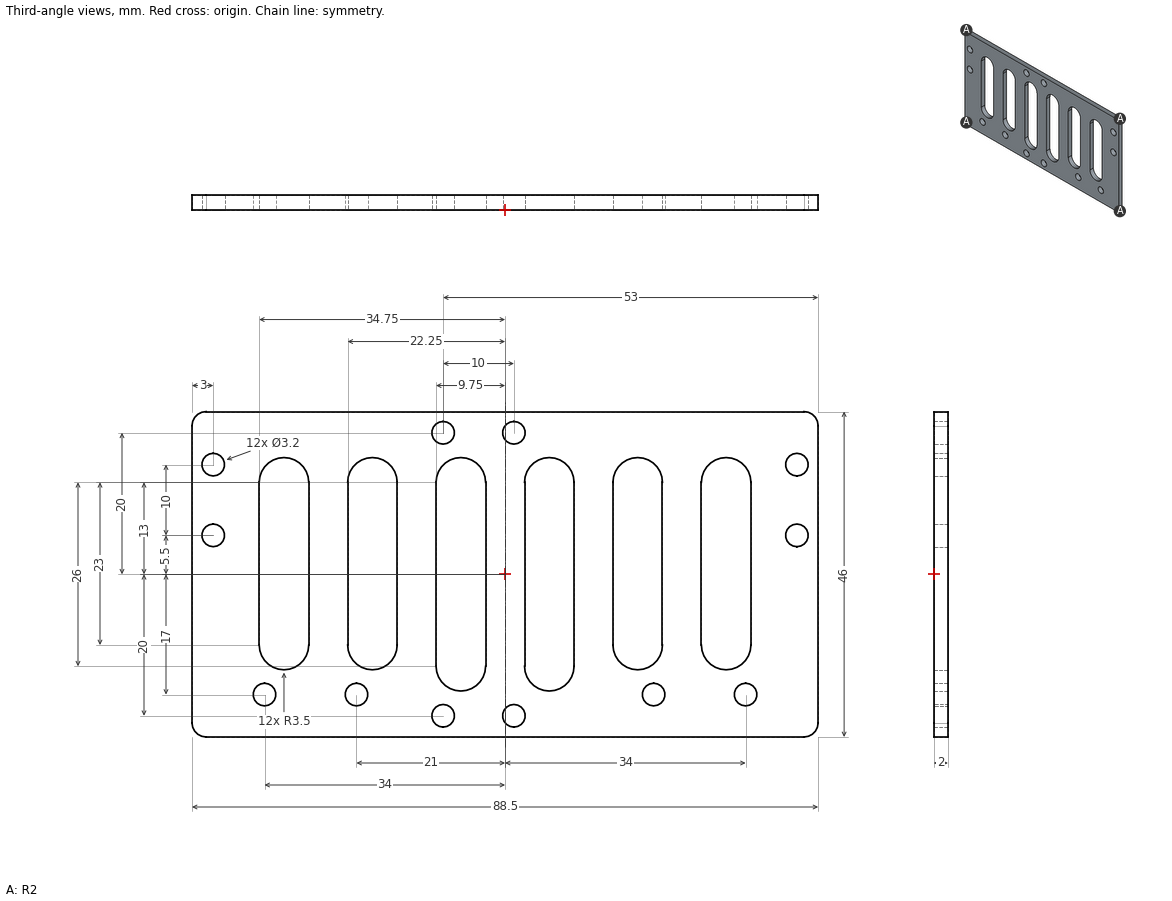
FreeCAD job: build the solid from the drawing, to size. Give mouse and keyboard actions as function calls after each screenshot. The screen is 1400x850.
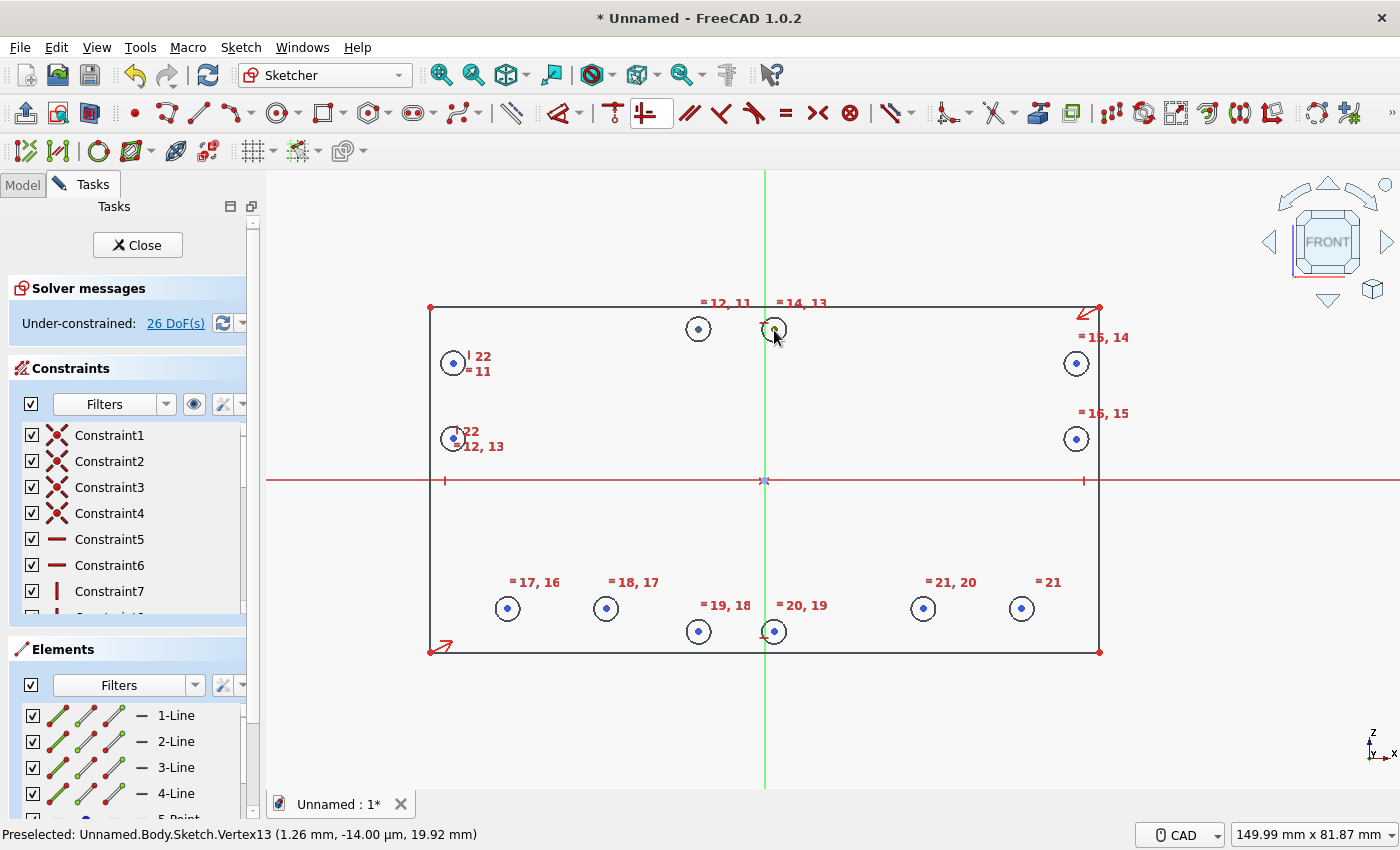
key(h)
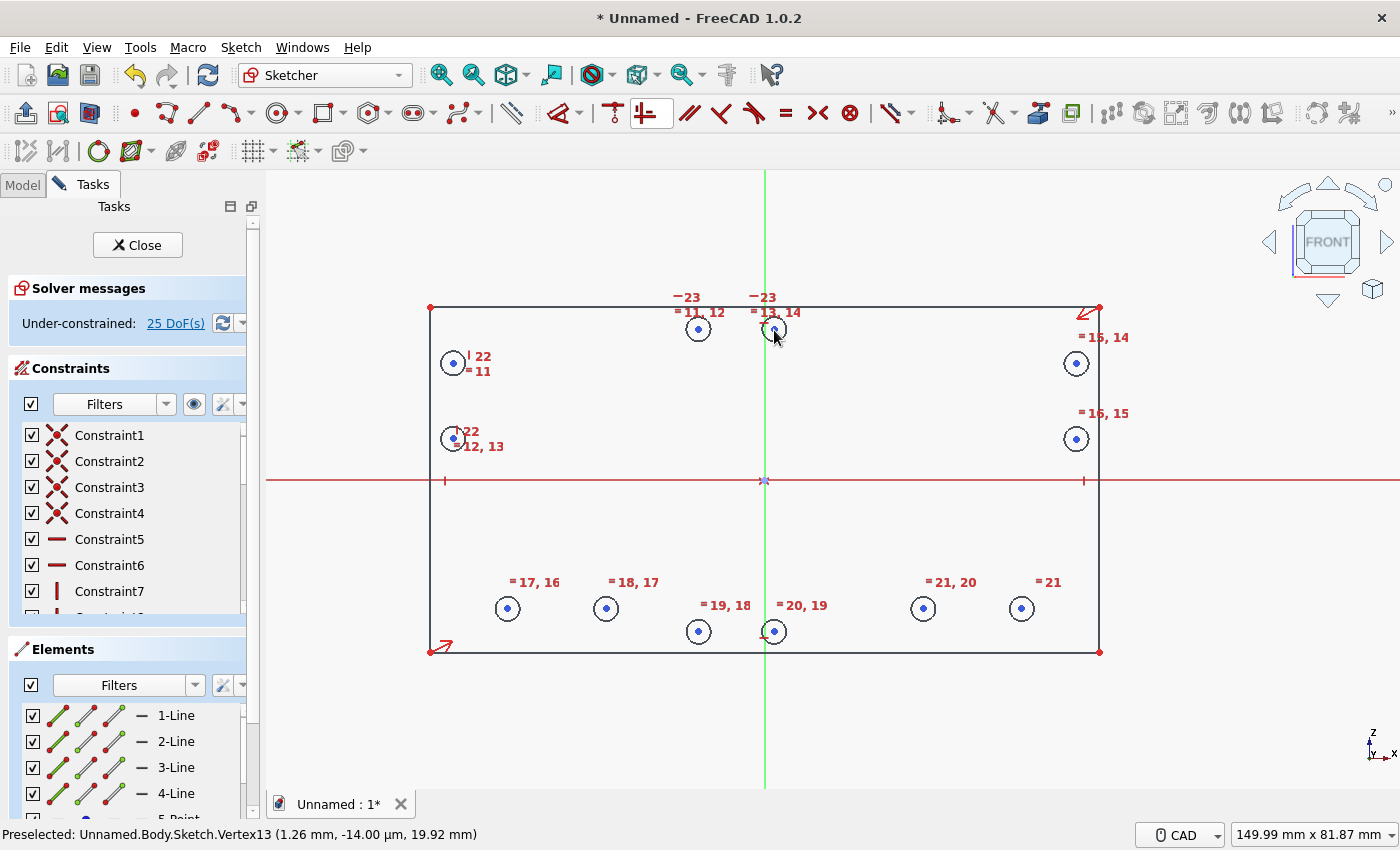
click(1076, 364)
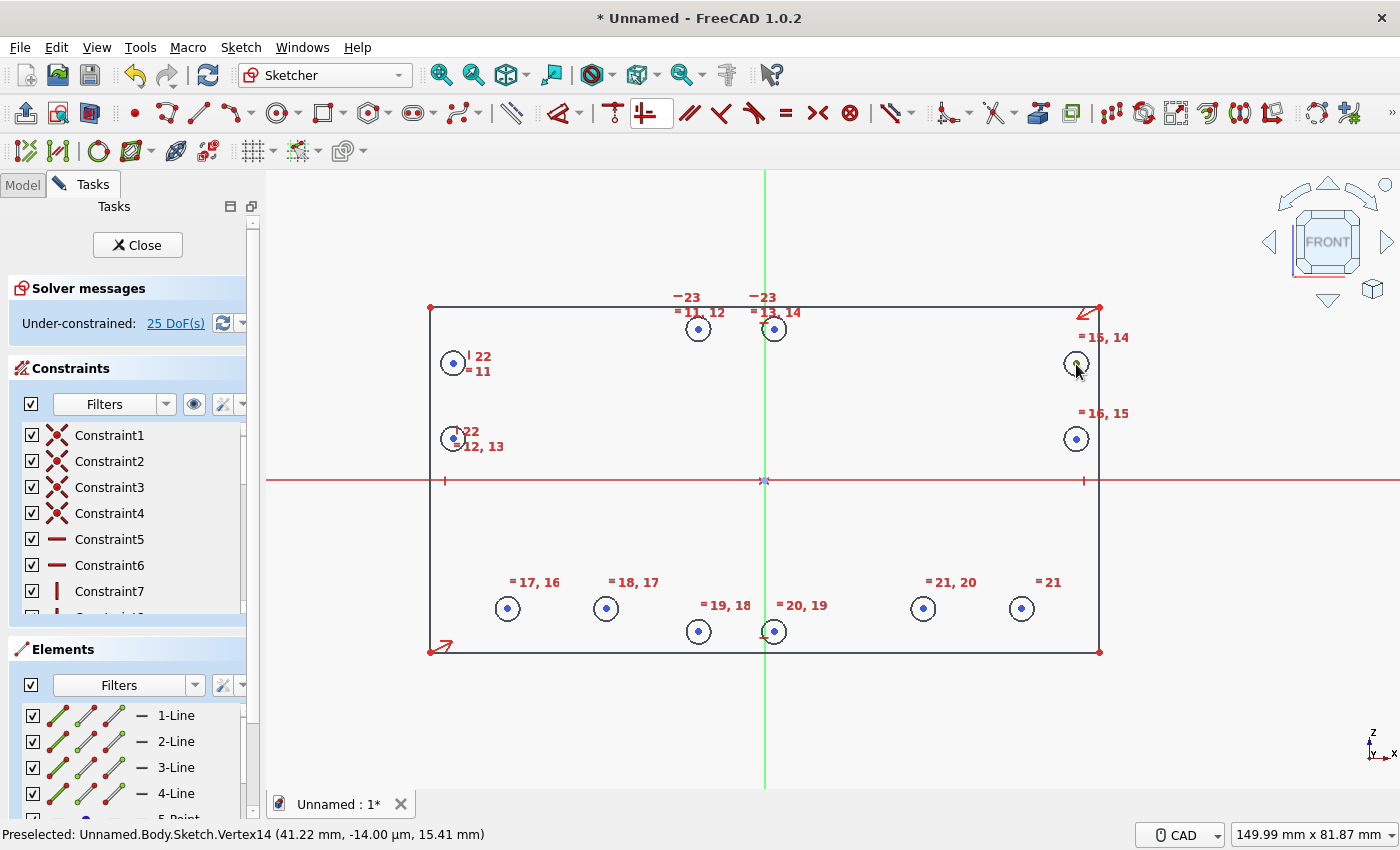
click(1076, 439)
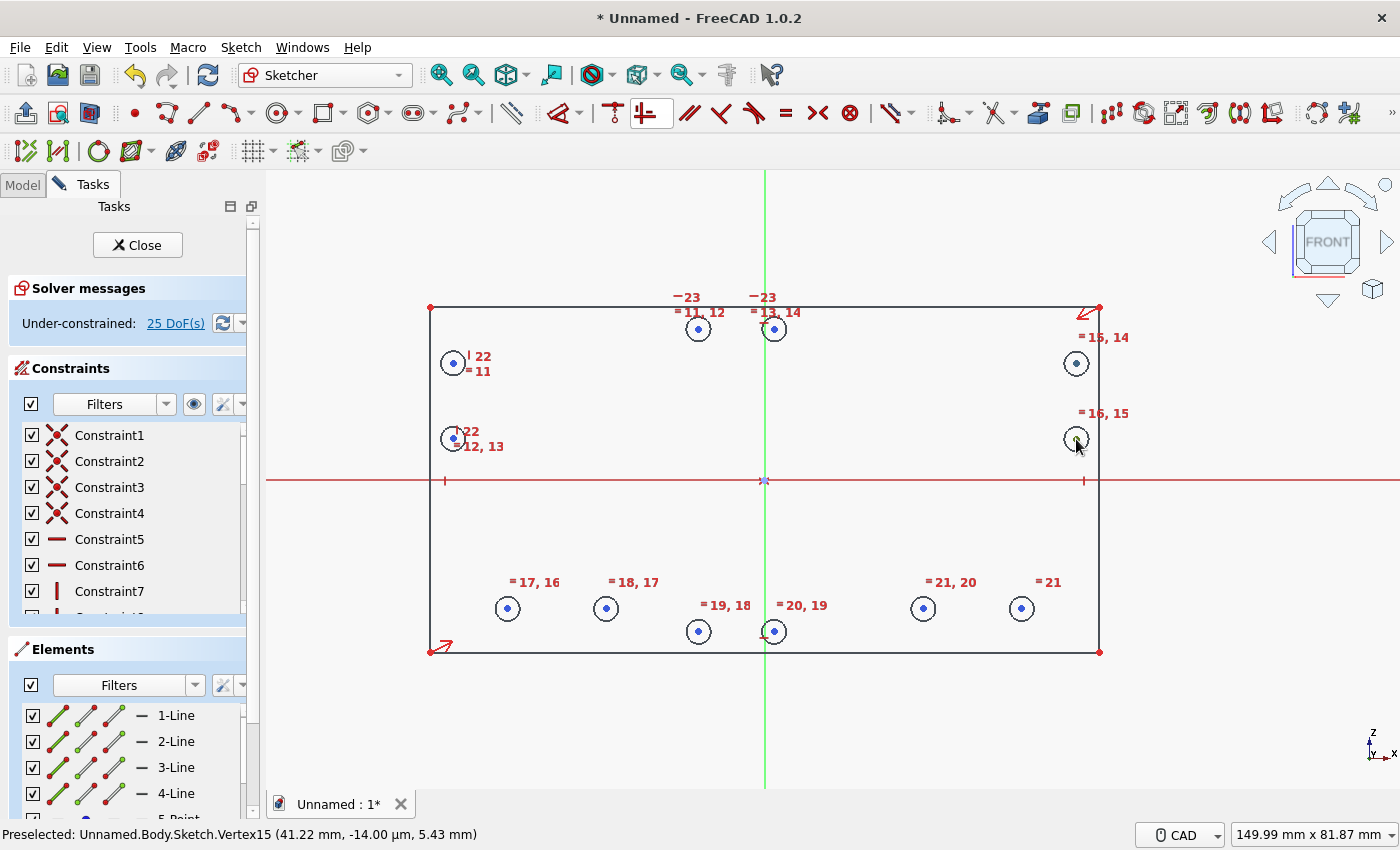
key(v)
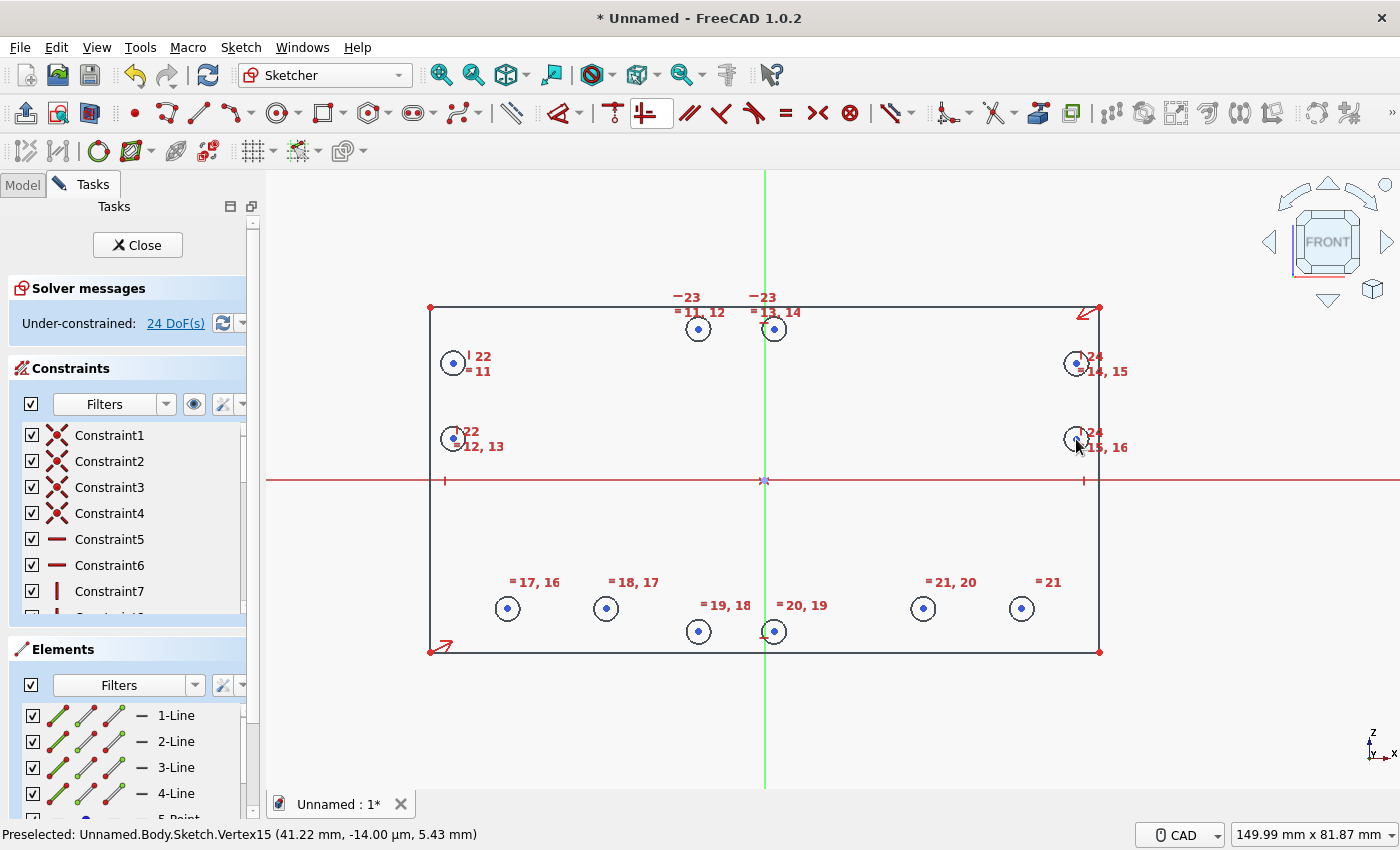
click(508, 609)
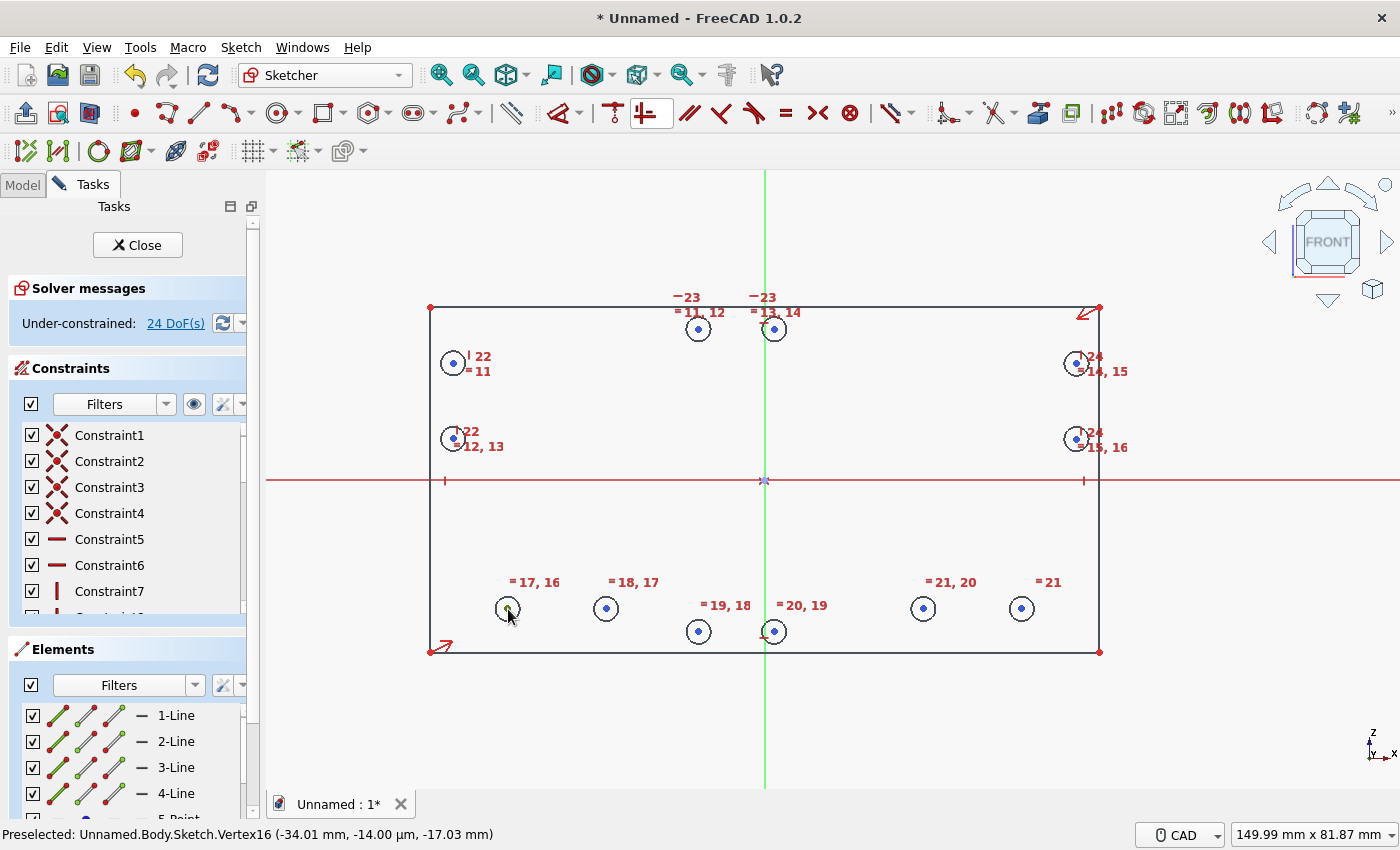
click(606, 609)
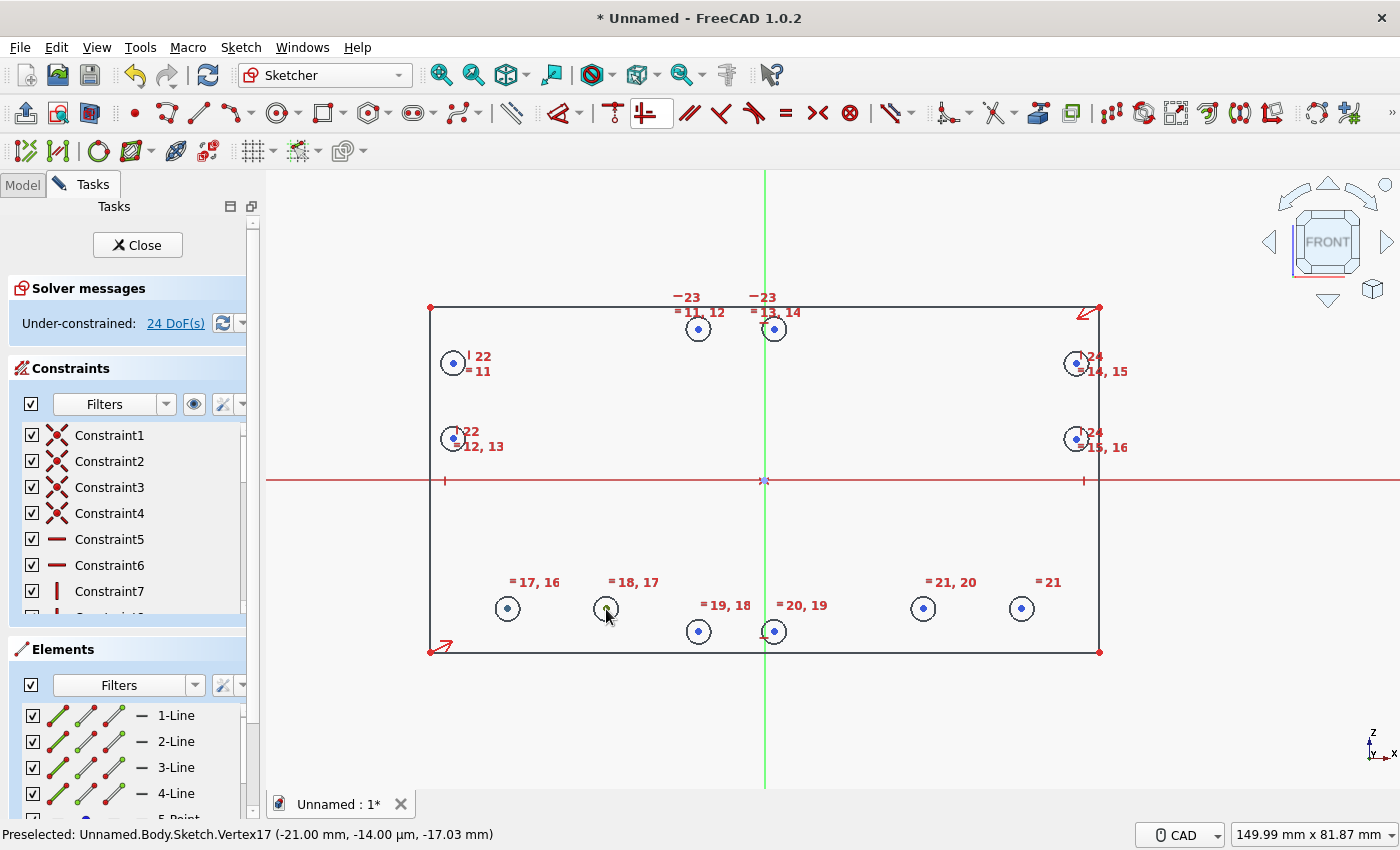
click(668, 114)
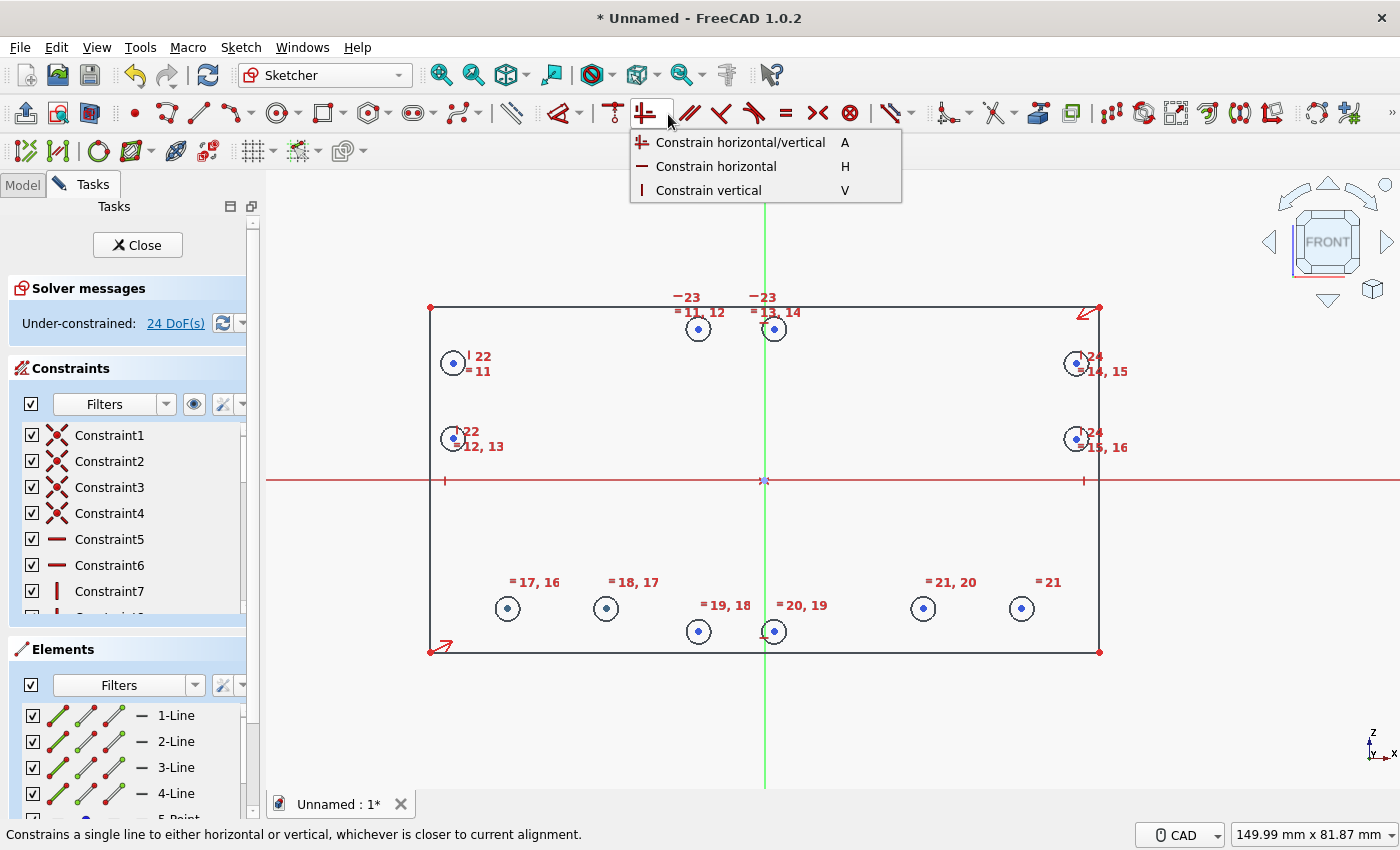
click(766, 166)